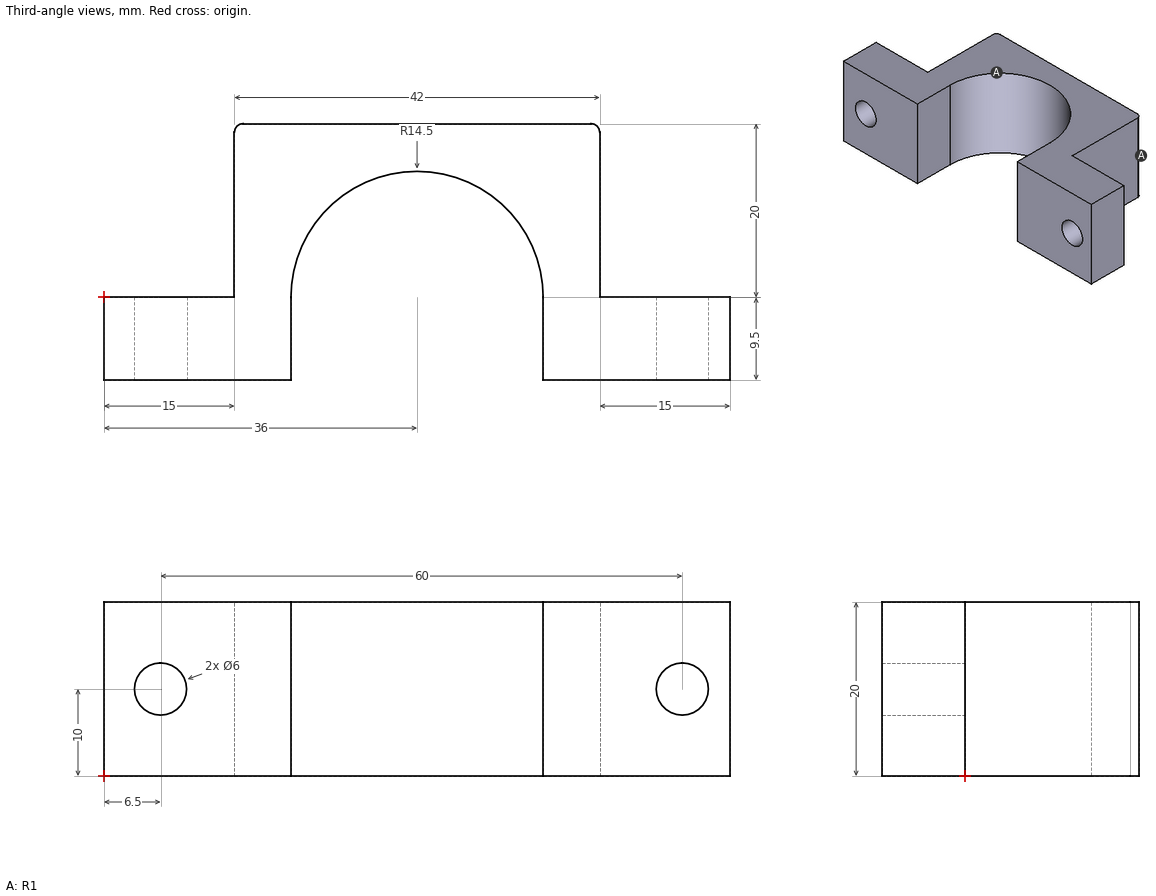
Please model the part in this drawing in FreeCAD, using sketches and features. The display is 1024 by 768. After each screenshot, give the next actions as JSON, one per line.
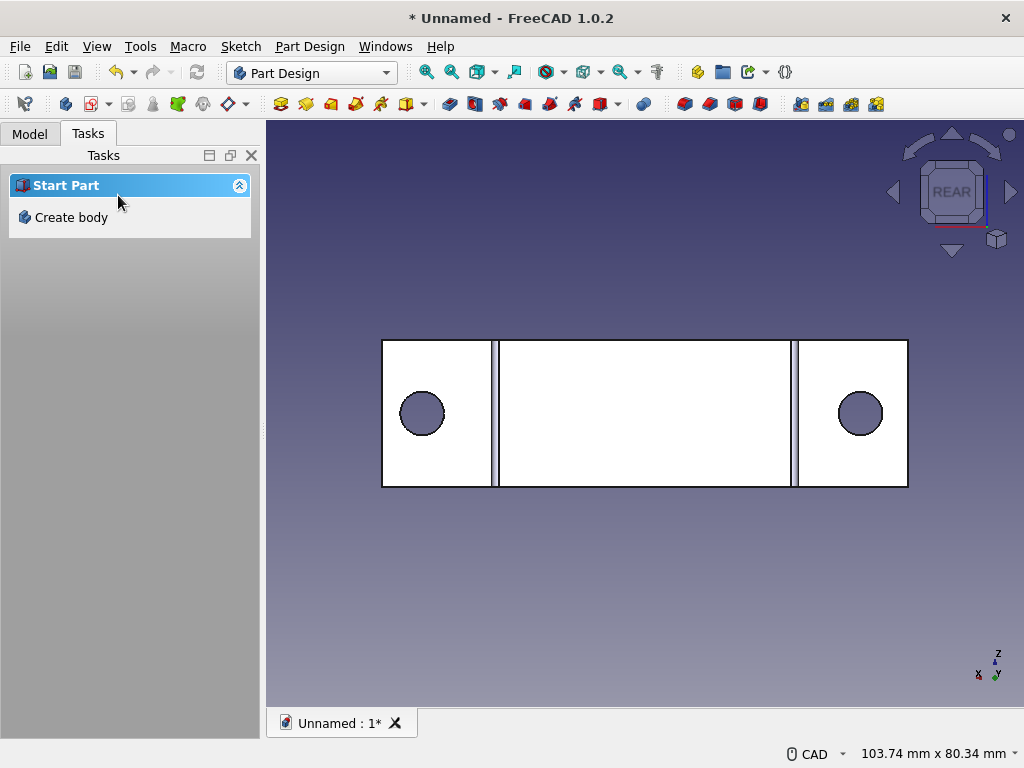
{"action": "key", "text": "0"}